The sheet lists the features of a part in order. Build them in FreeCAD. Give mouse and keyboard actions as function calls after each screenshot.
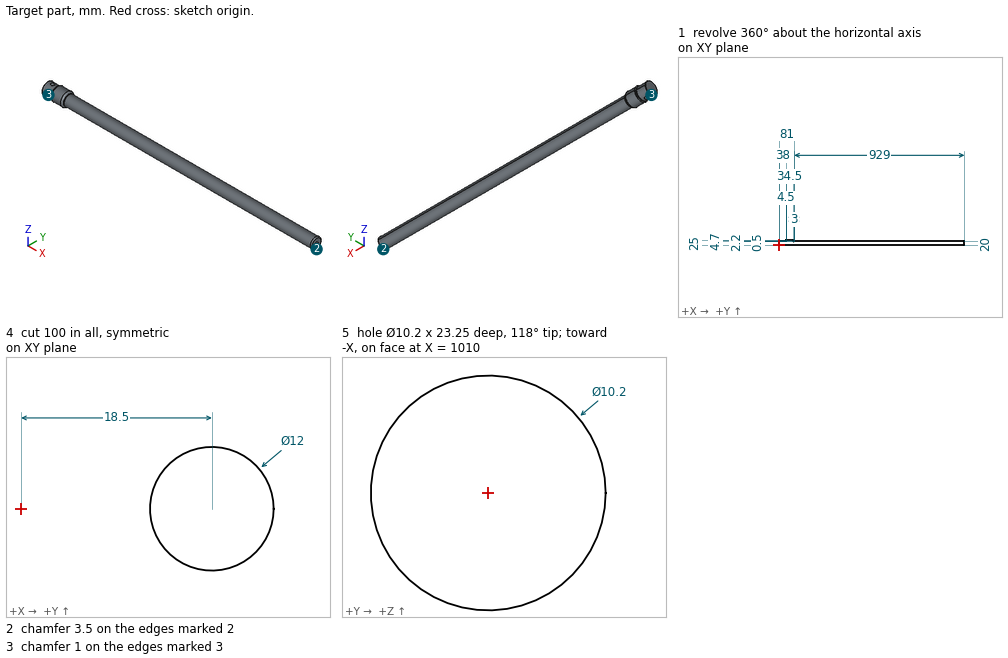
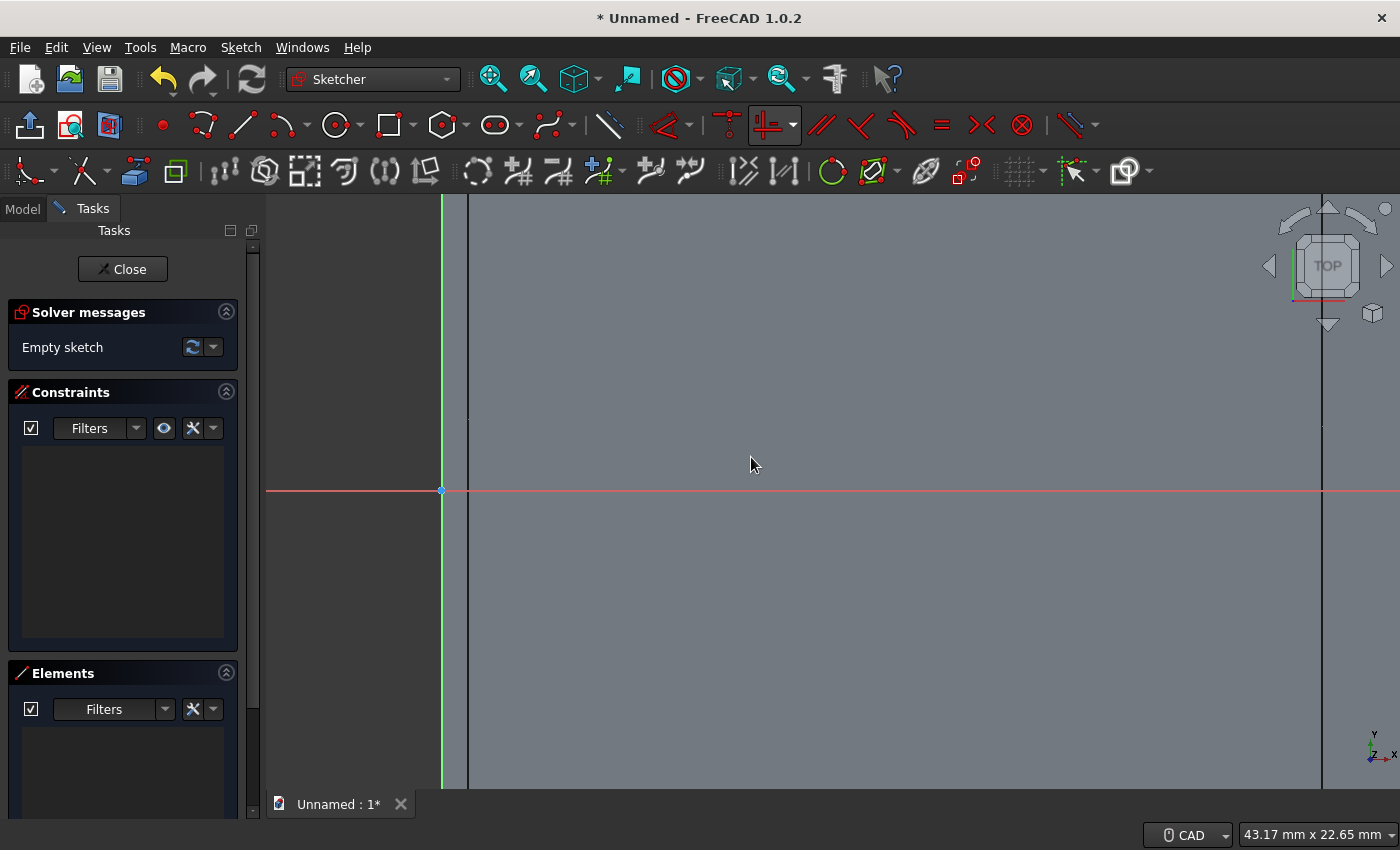
click(336, 126)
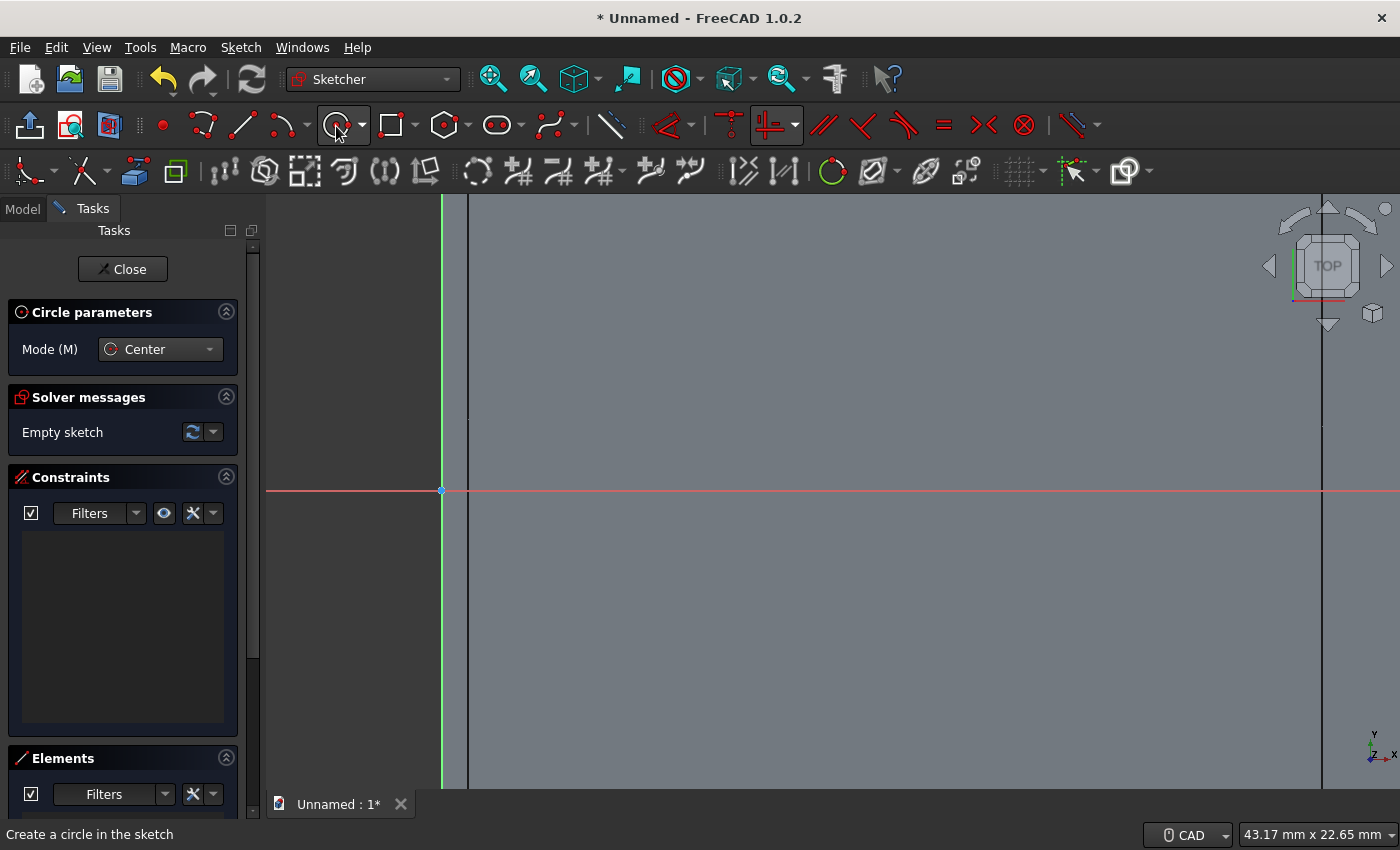
click(928, 491)
click(1039, 379)
key(Escape)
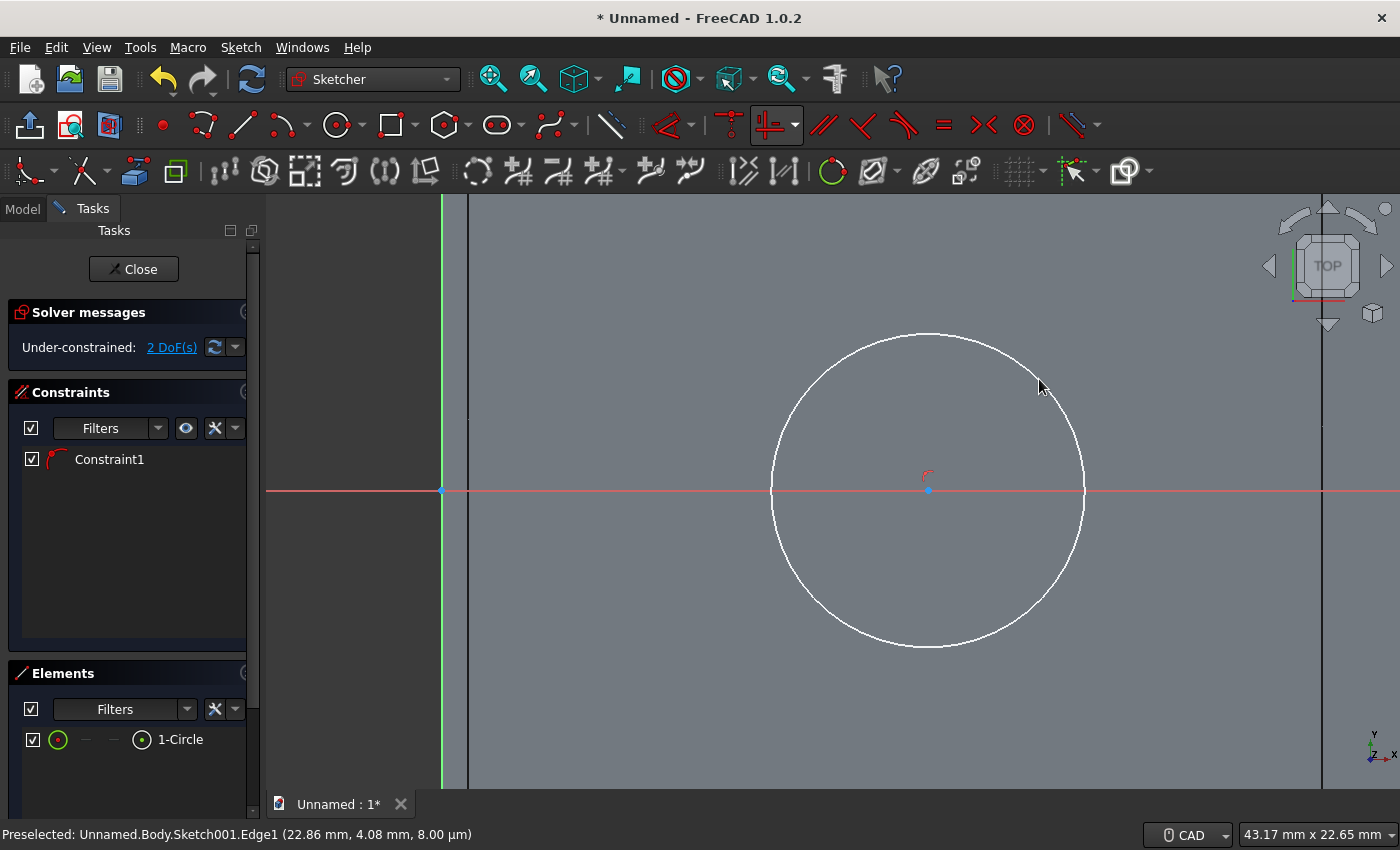
click(666, 126)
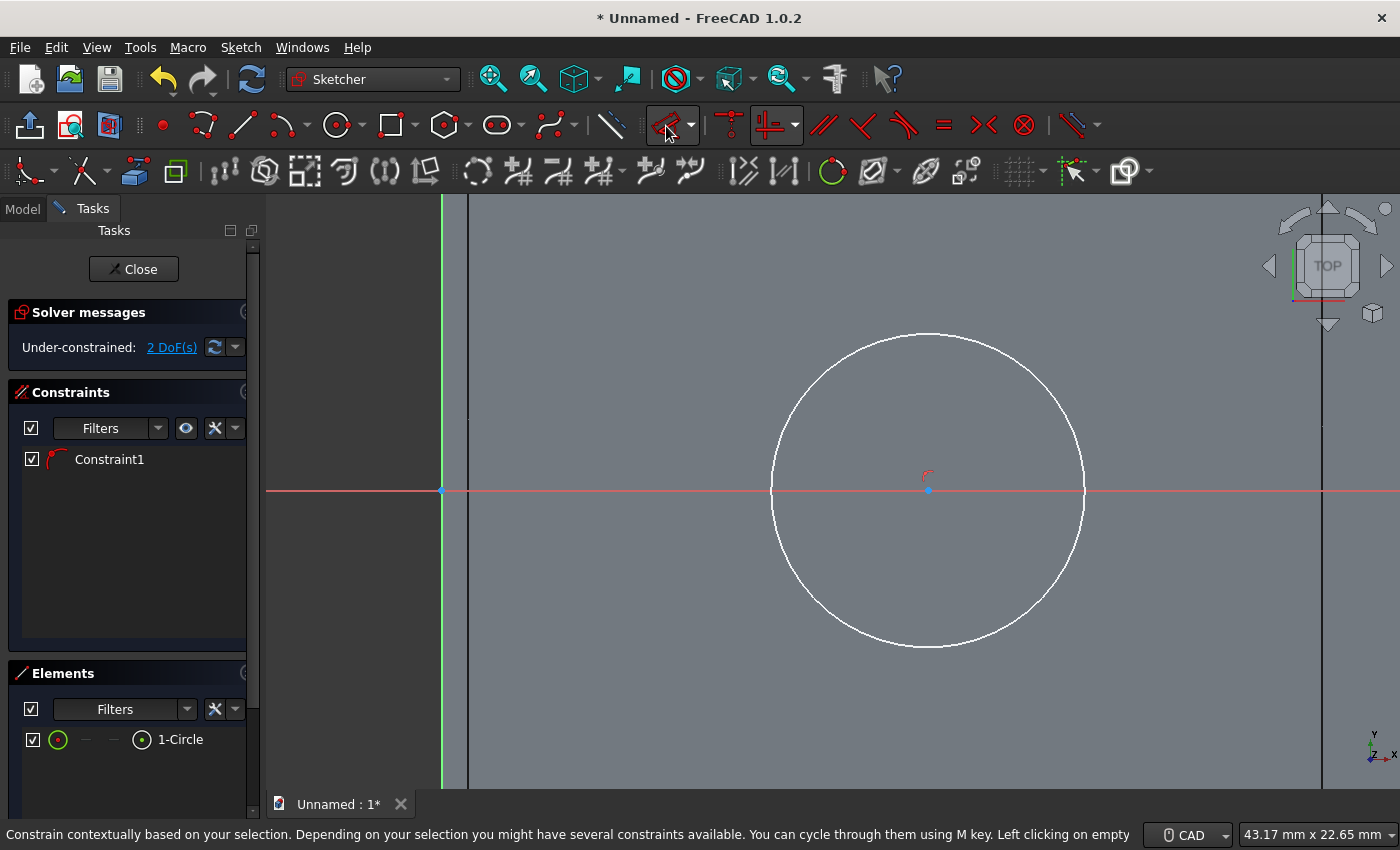
click(1039, 380)
click(1062, 357)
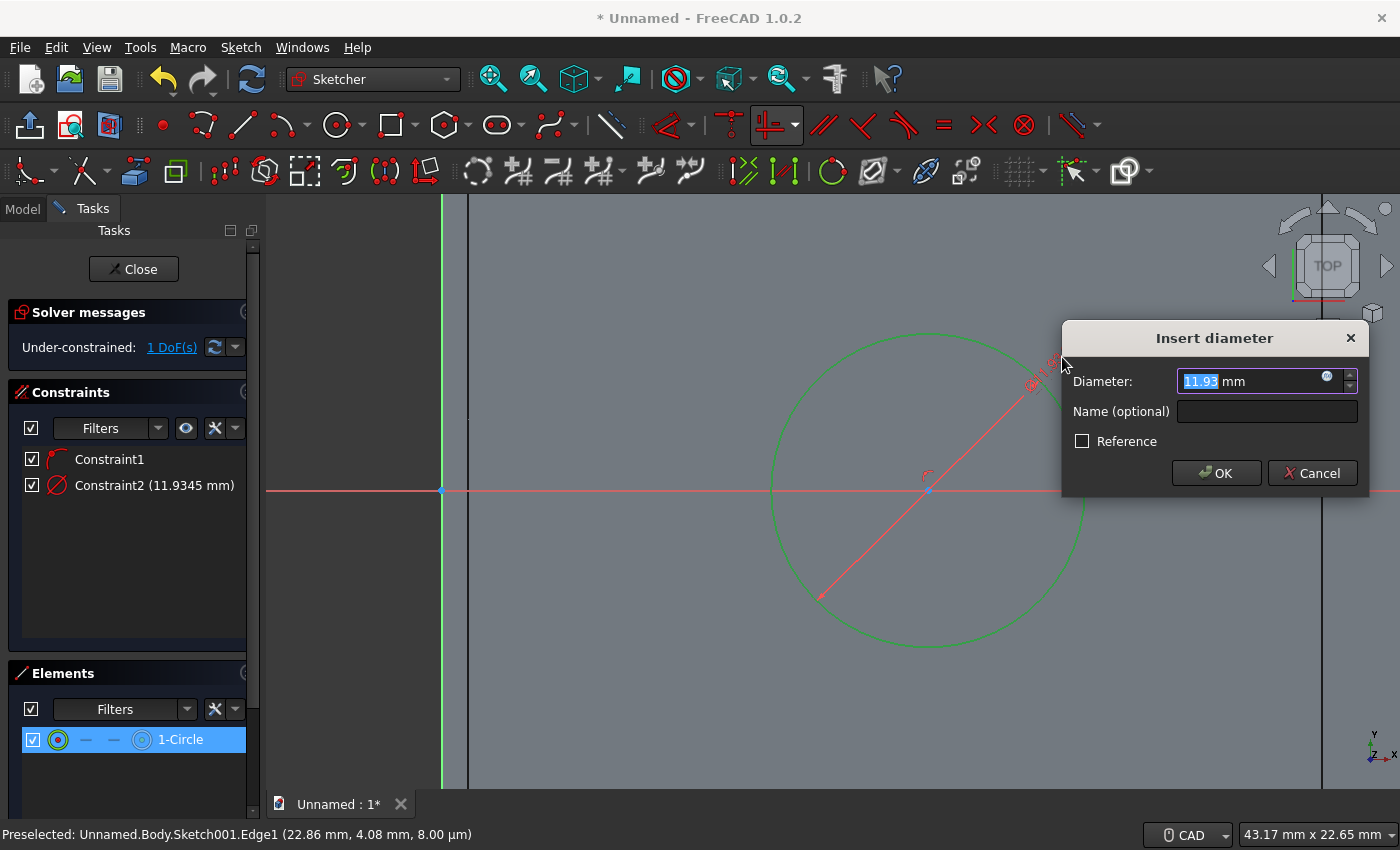
text(12)
key(Return)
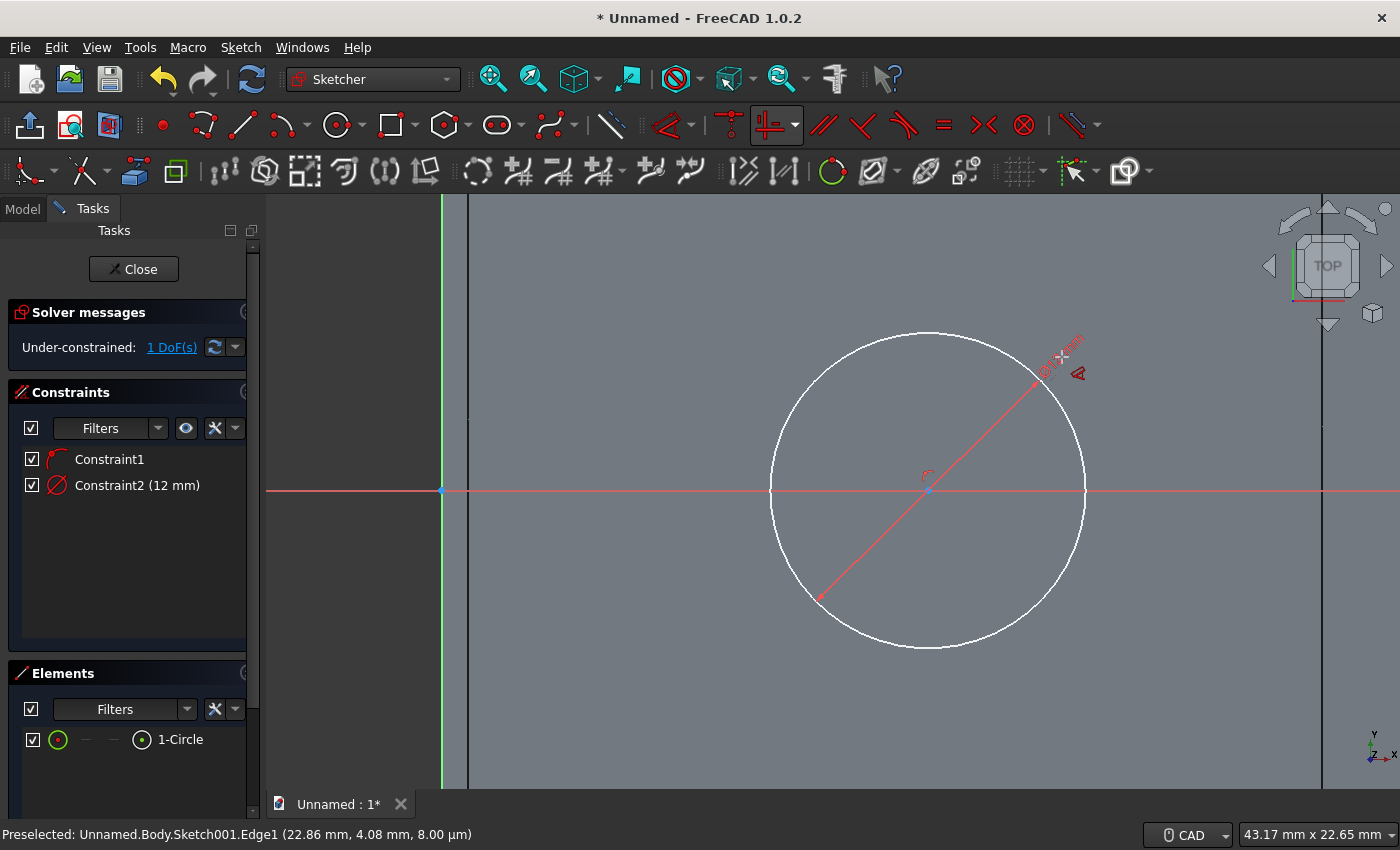
click(928, 491)
click(685, 525)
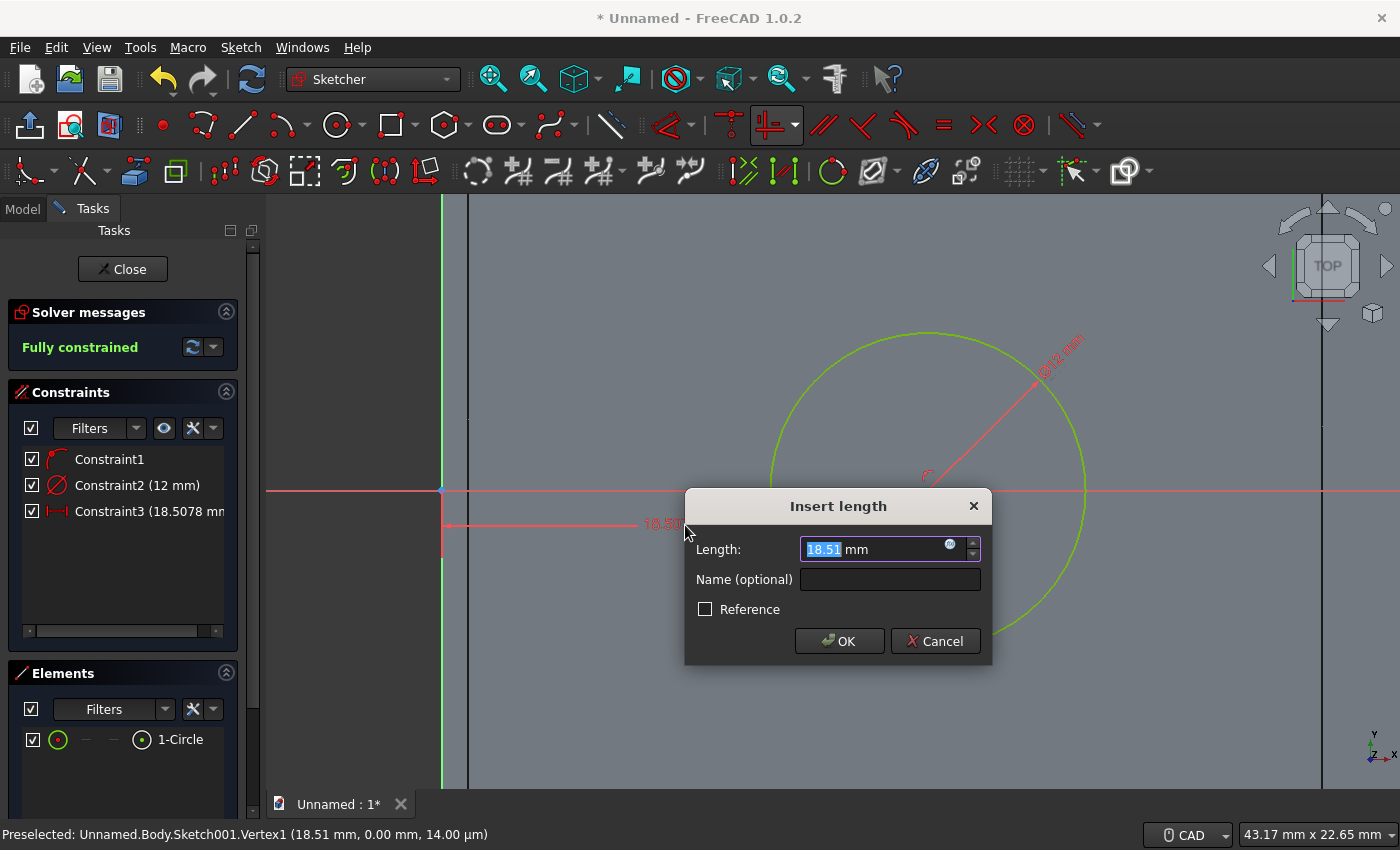
text(18.5)
key(Return)
key(Escape)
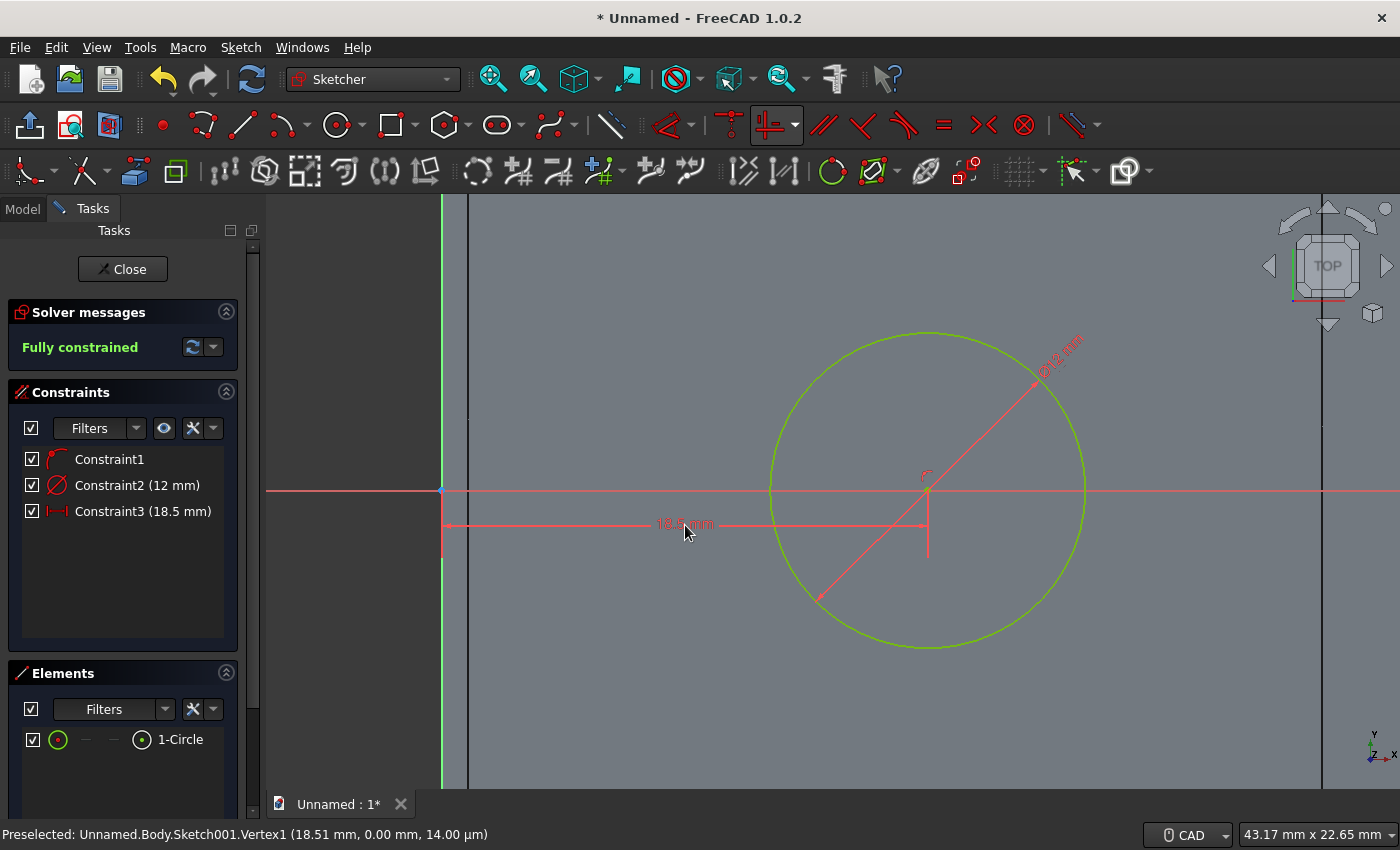
click(123, 269)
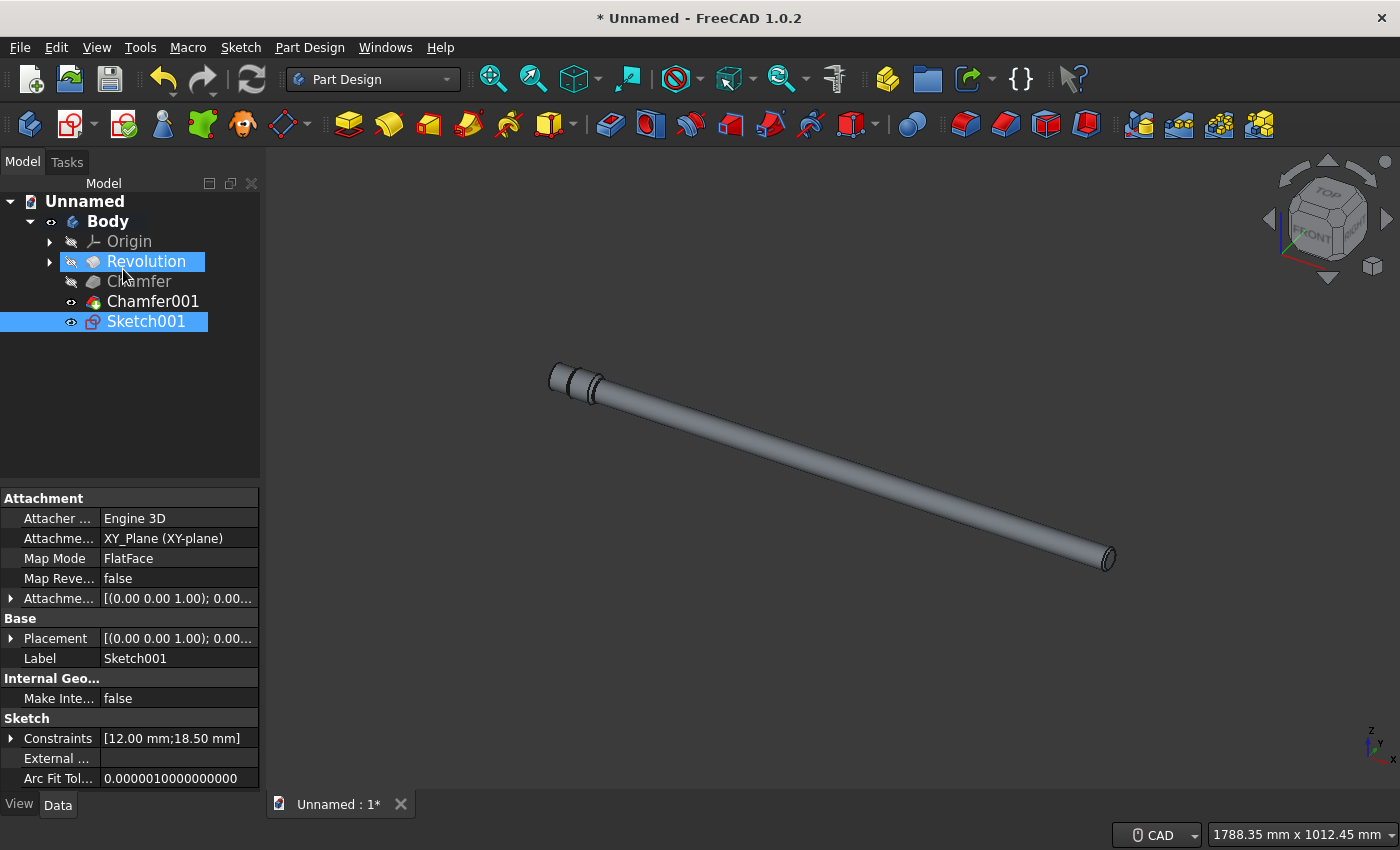
click(612, 124)